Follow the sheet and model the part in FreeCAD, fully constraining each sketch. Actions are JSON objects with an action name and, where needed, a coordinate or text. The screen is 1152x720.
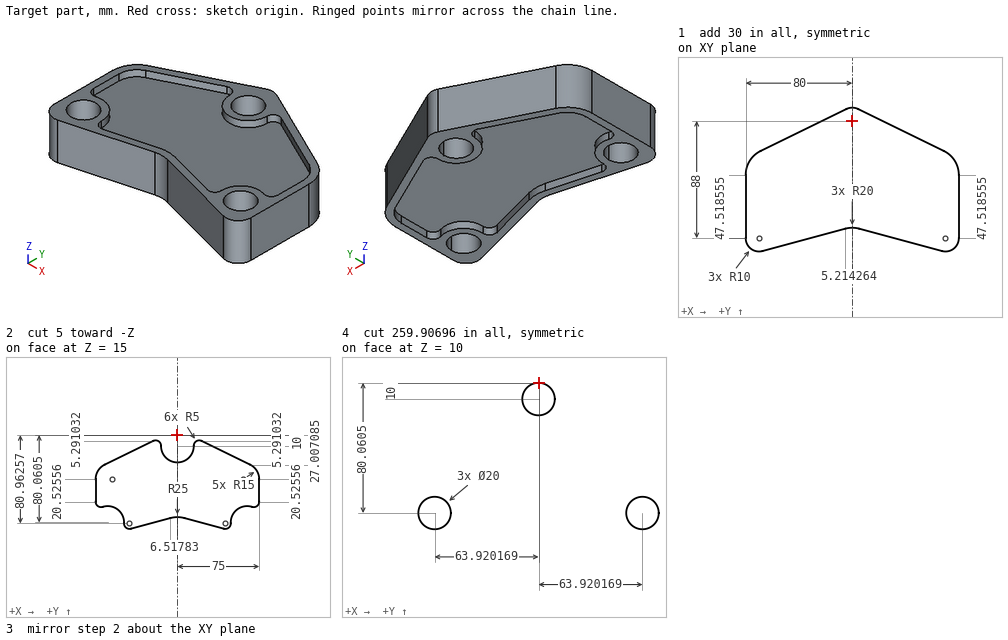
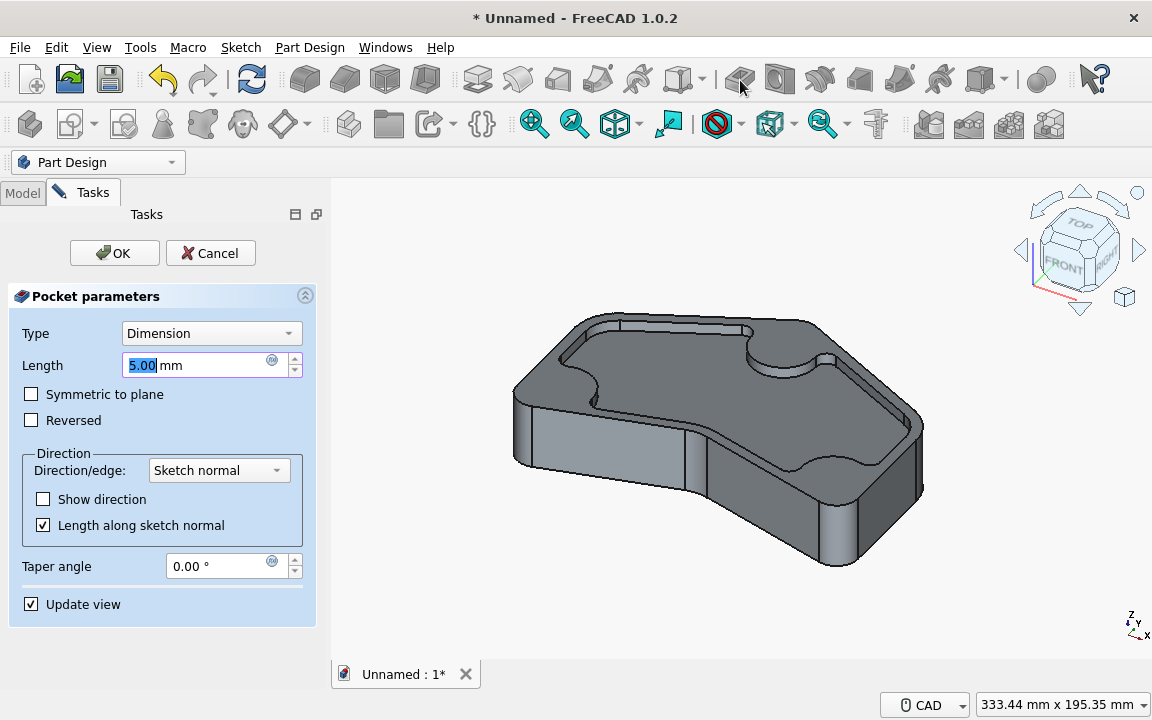
{"action": "type", "text": "259.90696"}
{"action": "key", "text": "Tab"}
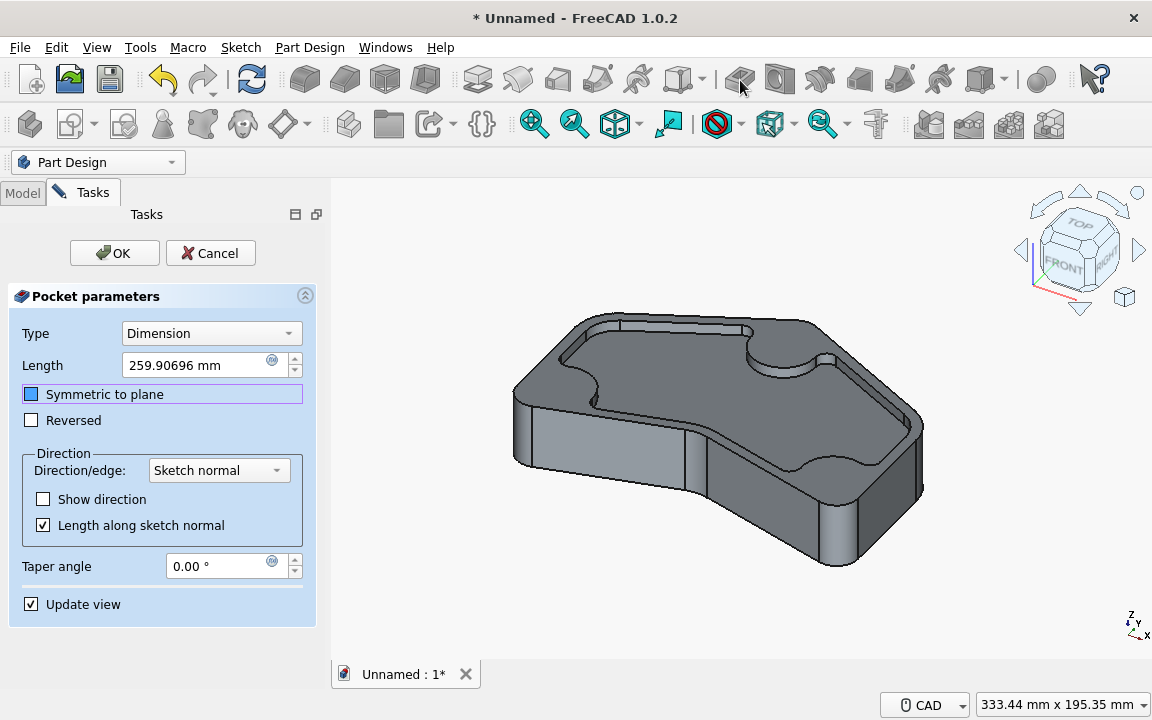
{"action": "left_click", "coordinate": [30, 394]}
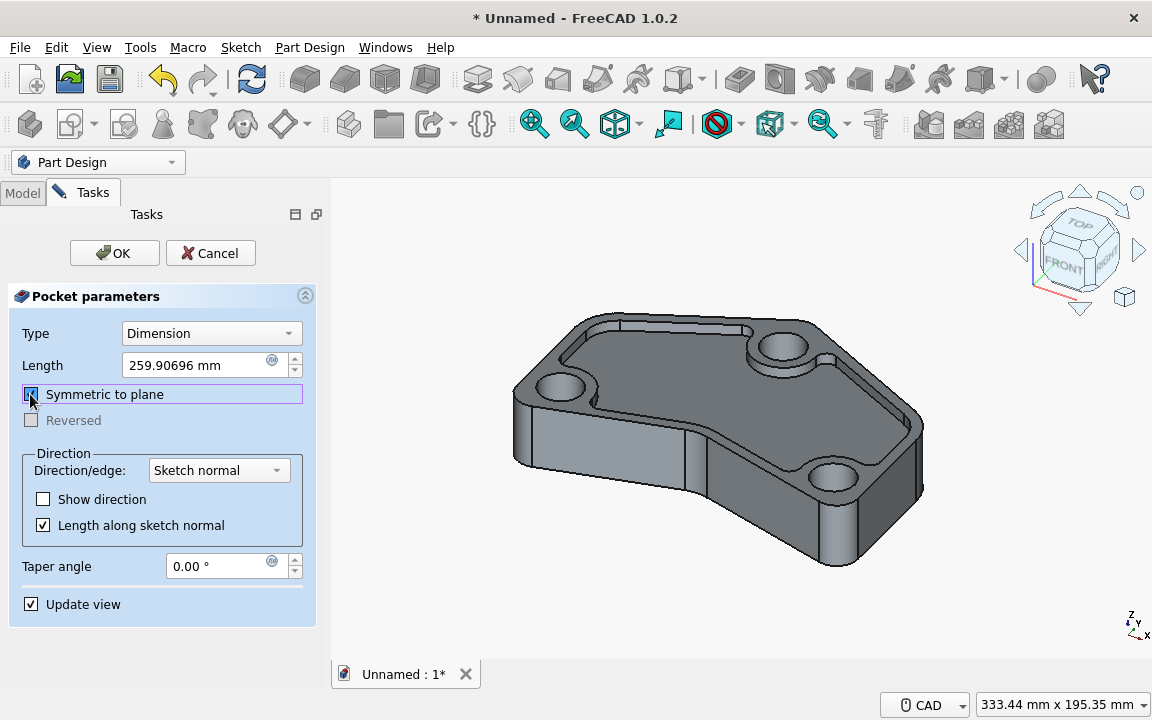
{"action": "left_click", "coordinate": [115, 253]}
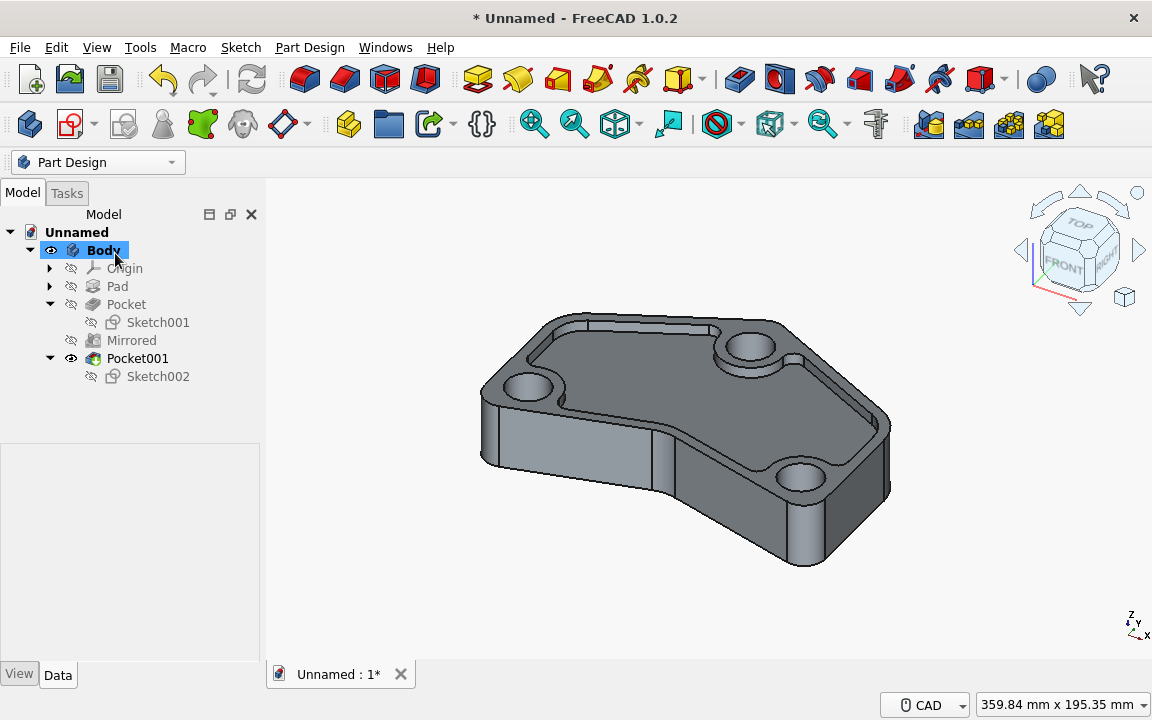
{"action": "key", "text": "0"}